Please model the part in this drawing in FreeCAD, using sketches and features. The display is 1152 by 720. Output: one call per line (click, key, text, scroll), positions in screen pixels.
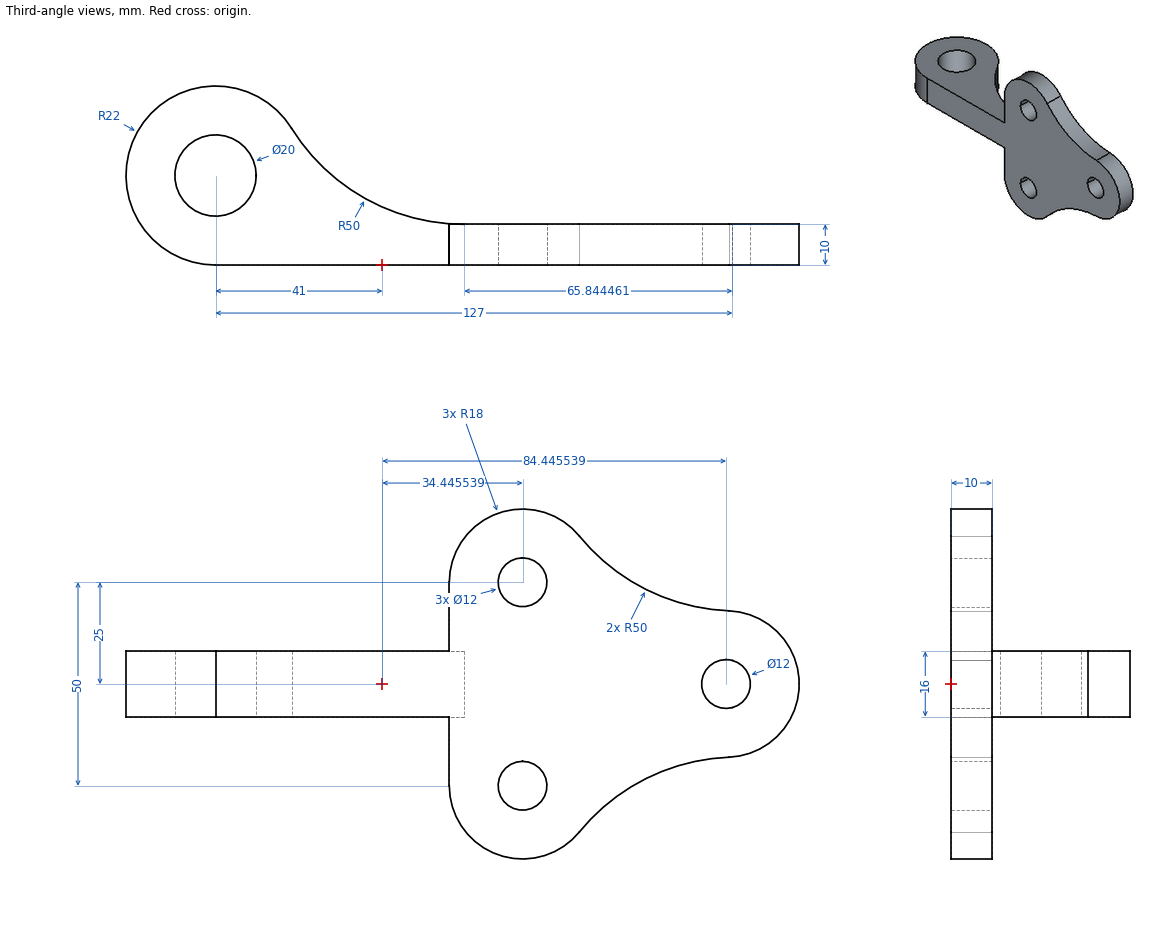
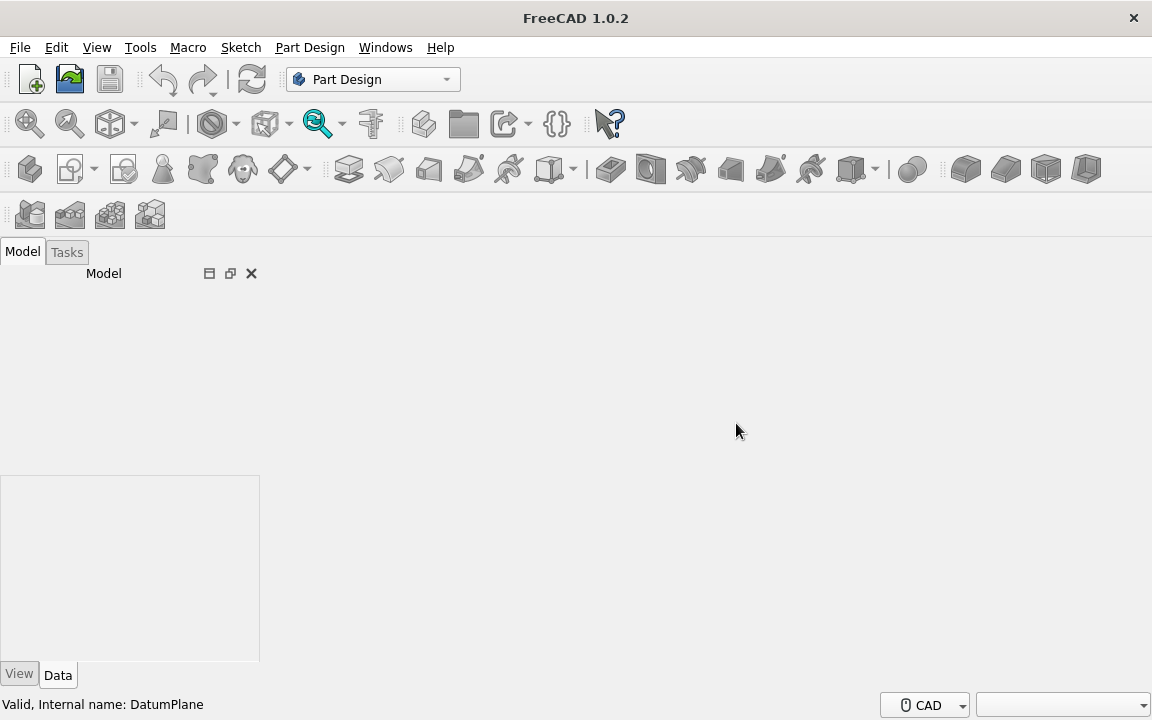
key(ctrl+n)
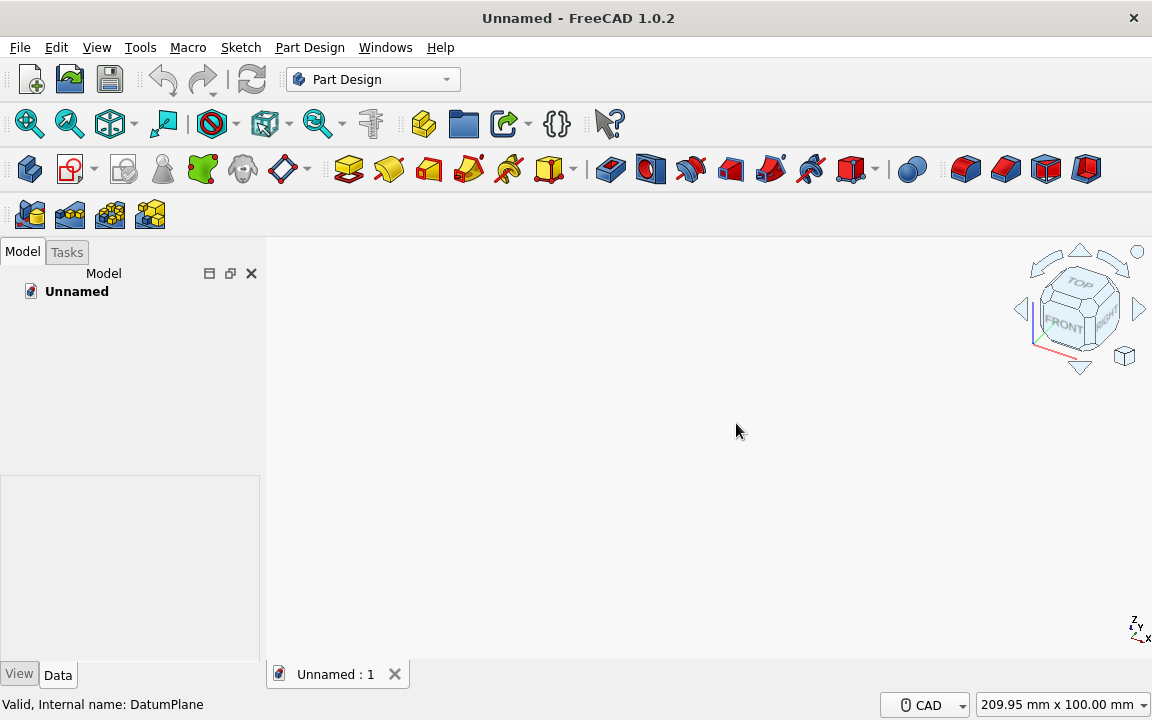
click(70, 170)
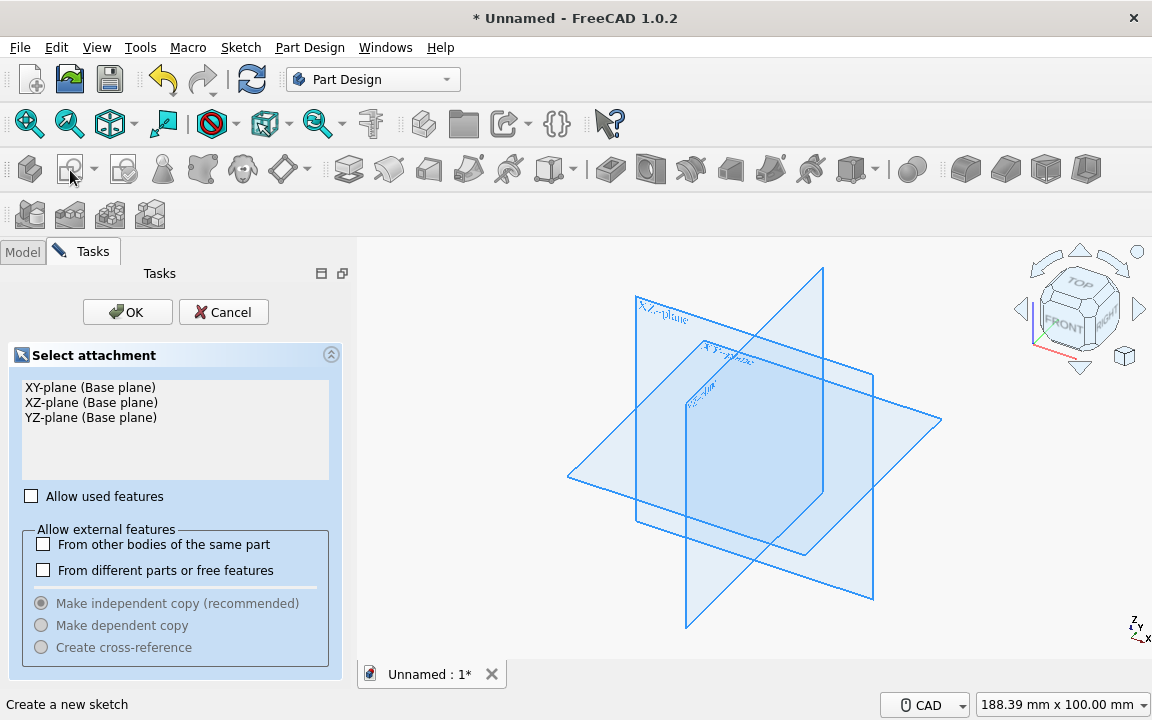
click(82, 388)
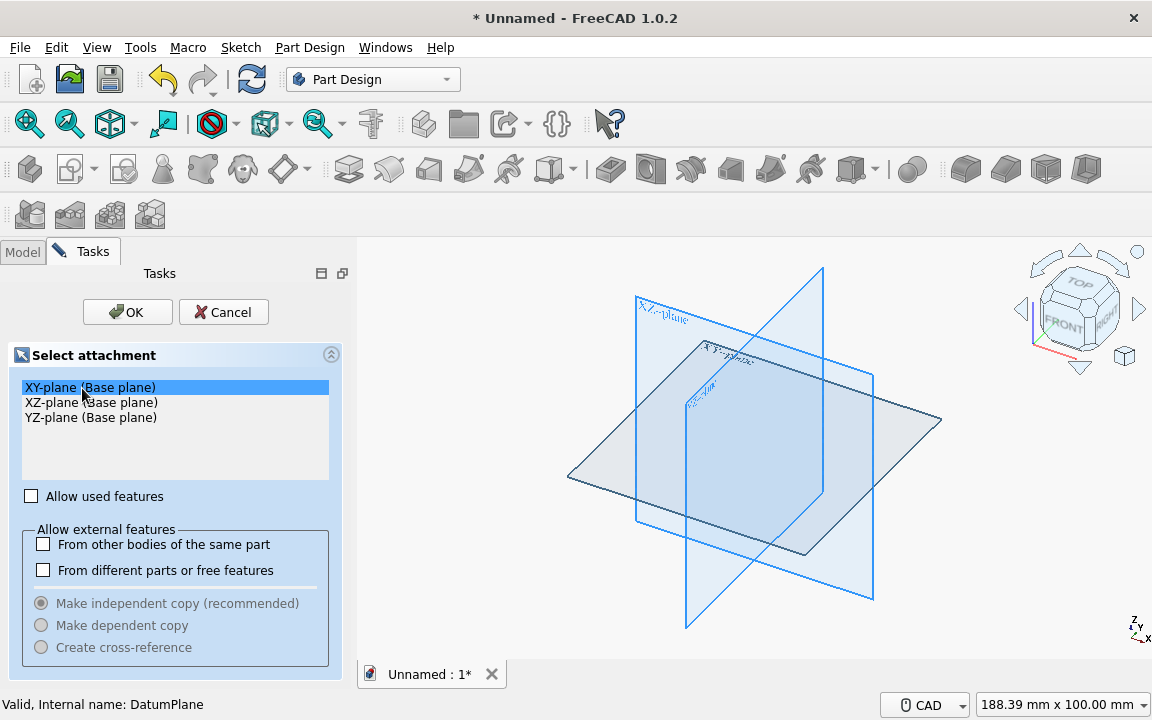
click(128, 312)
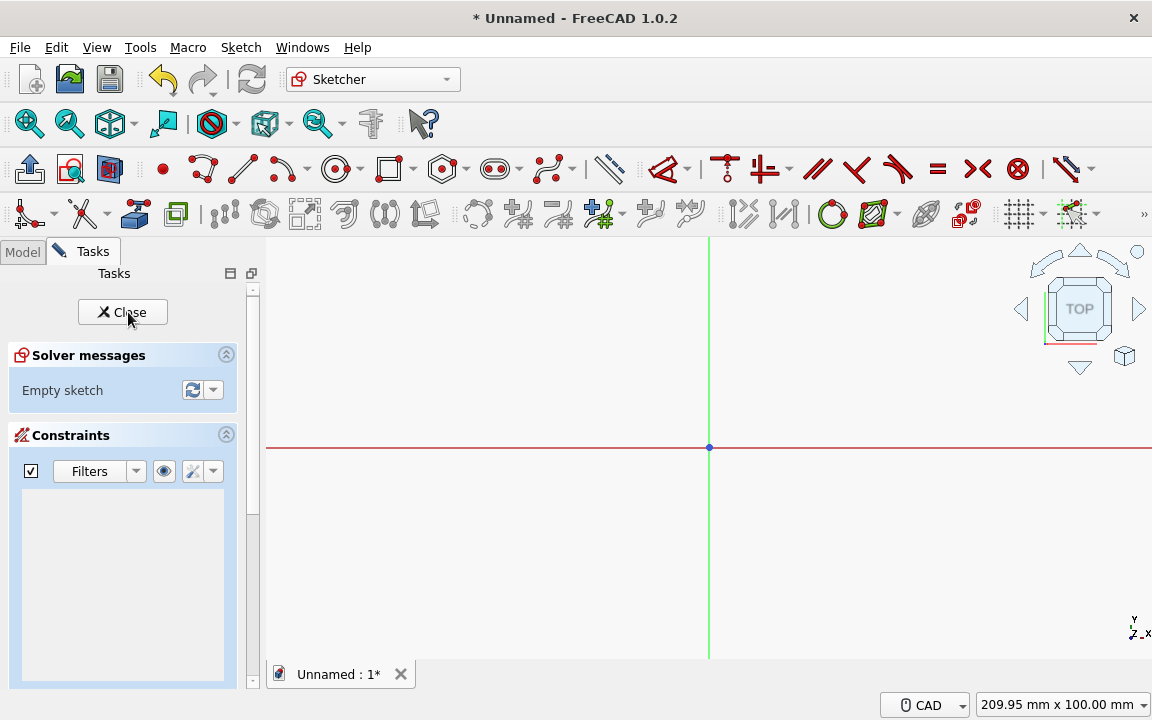
scroll(294, 631, down, 1)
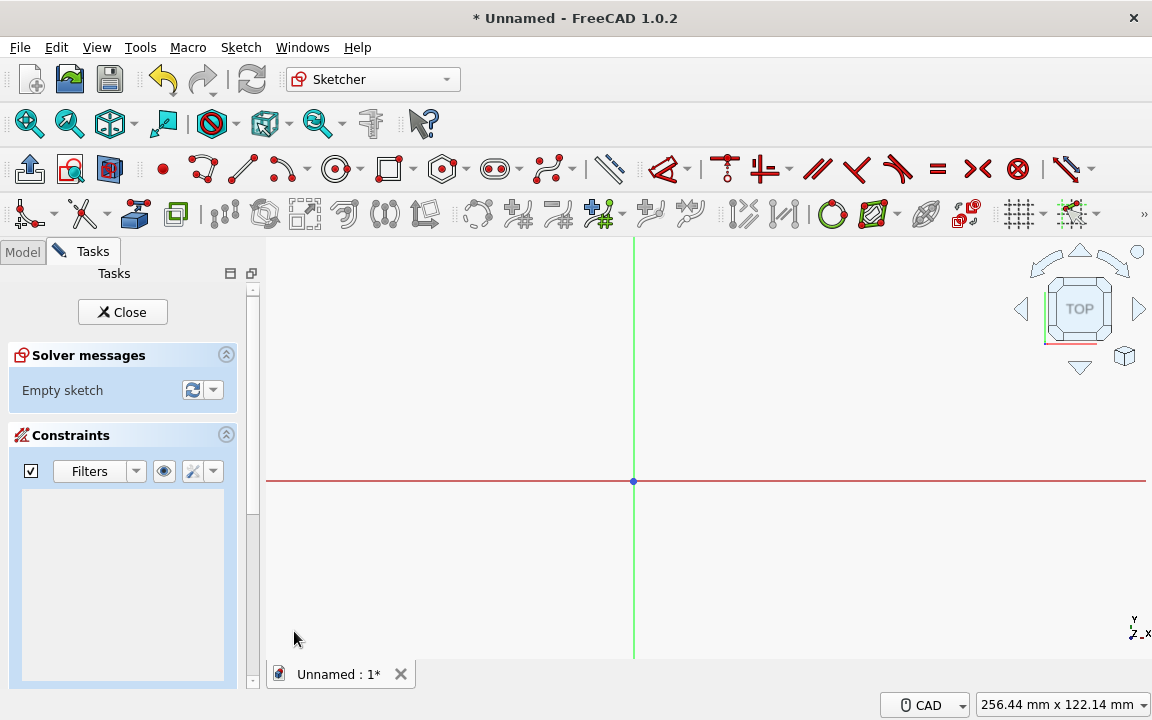
key(g)
key(m)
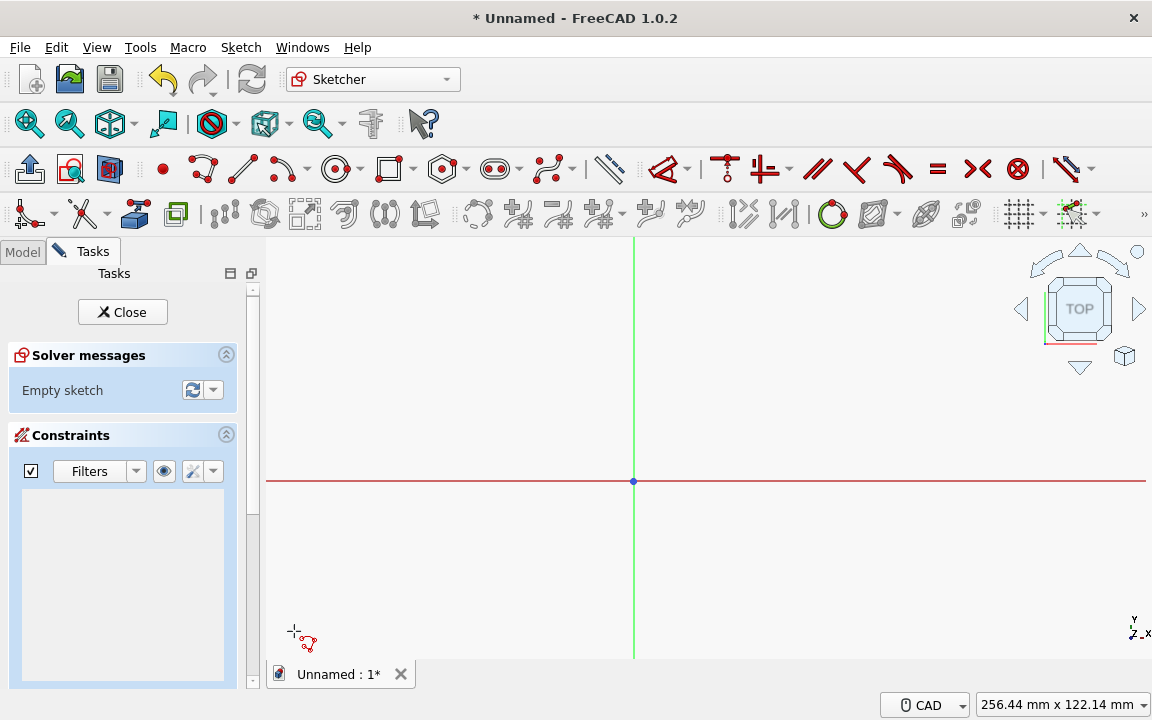
click(492, 481)
click(931, 472)
click(931, 447)
click(703, 447)
right_click(703, 447)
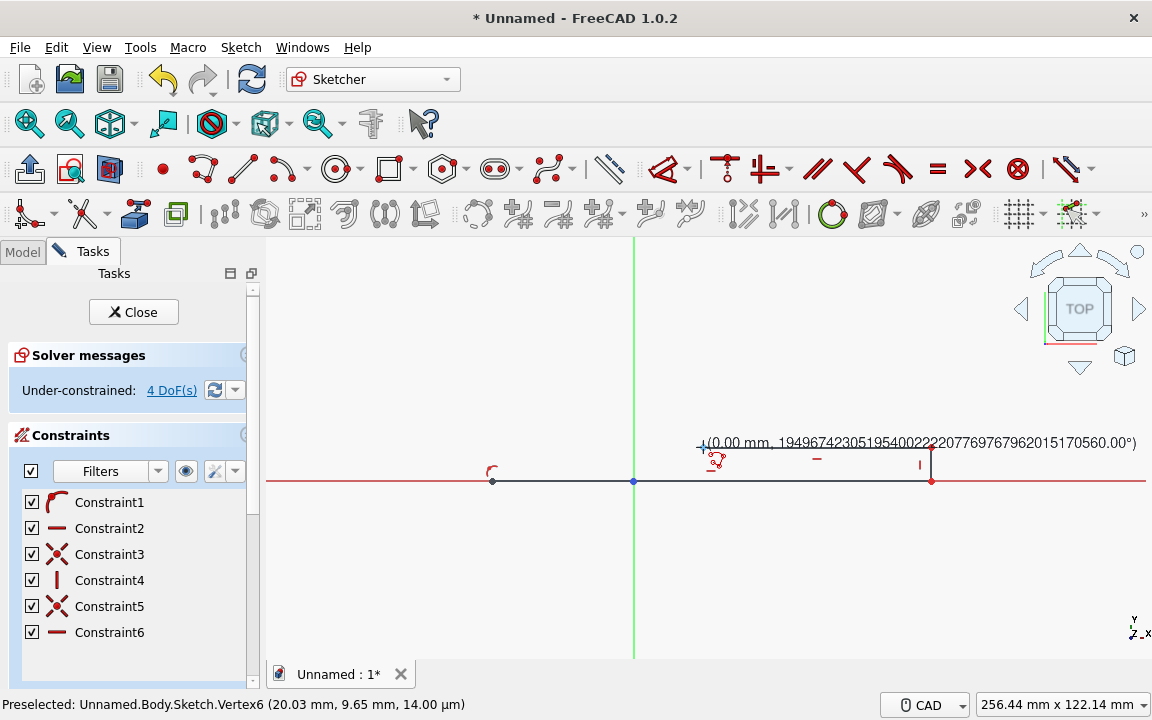
key(g)
key(3)
key(a)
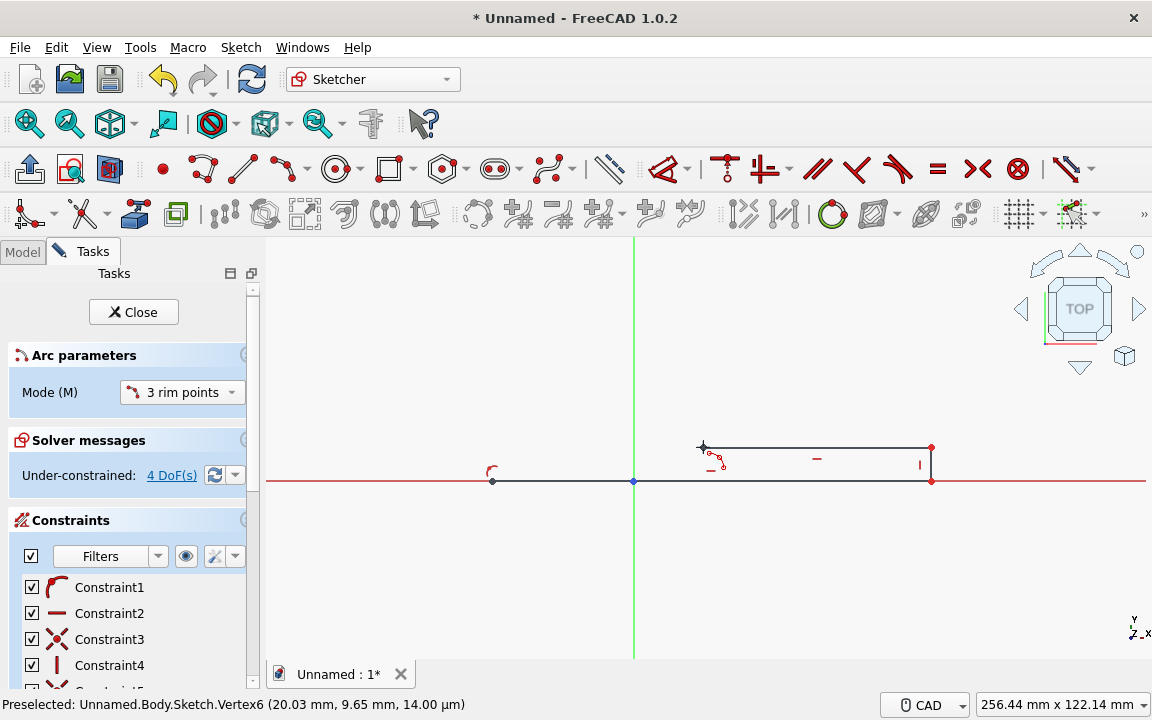
click(703, 448)
click(557, 365)
click(619, 425)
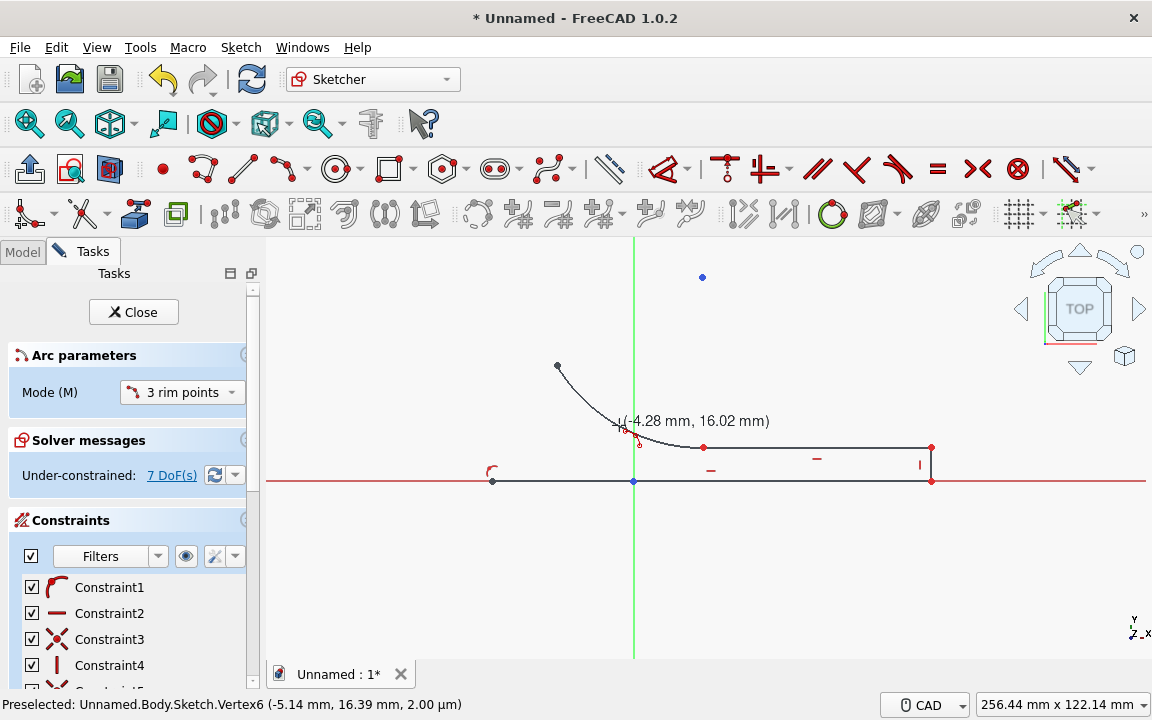
click(557, 366)
click(492, 481)
click(426, 368)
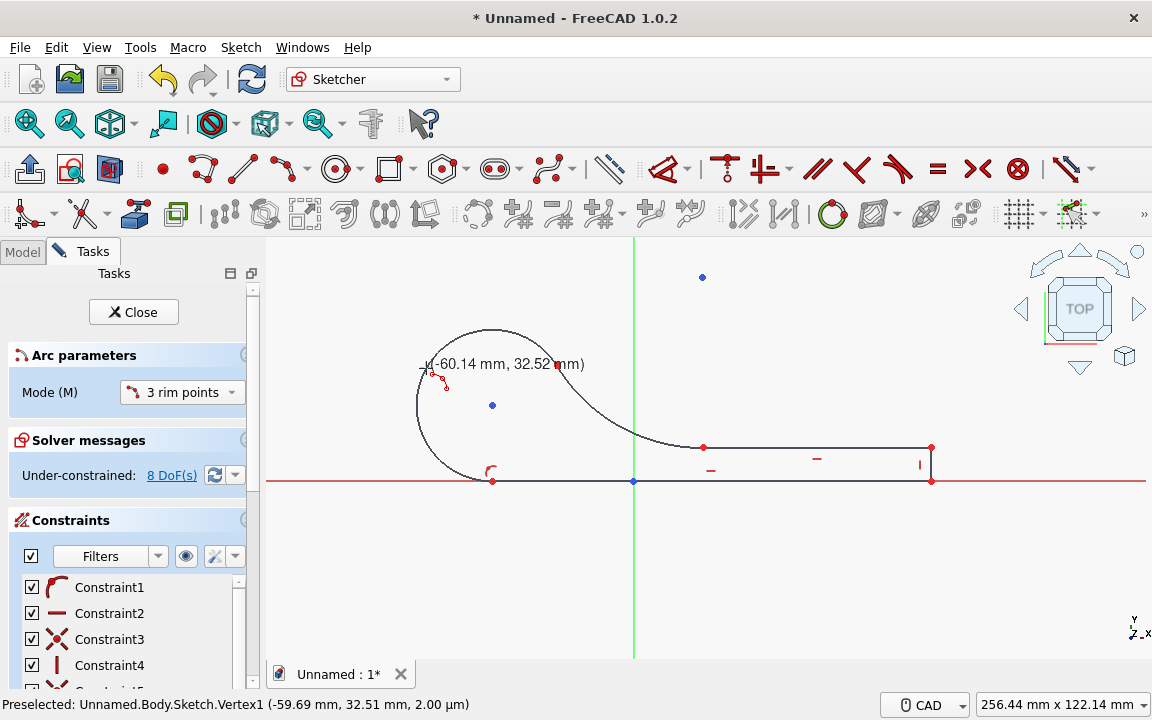
key(g)
key(c)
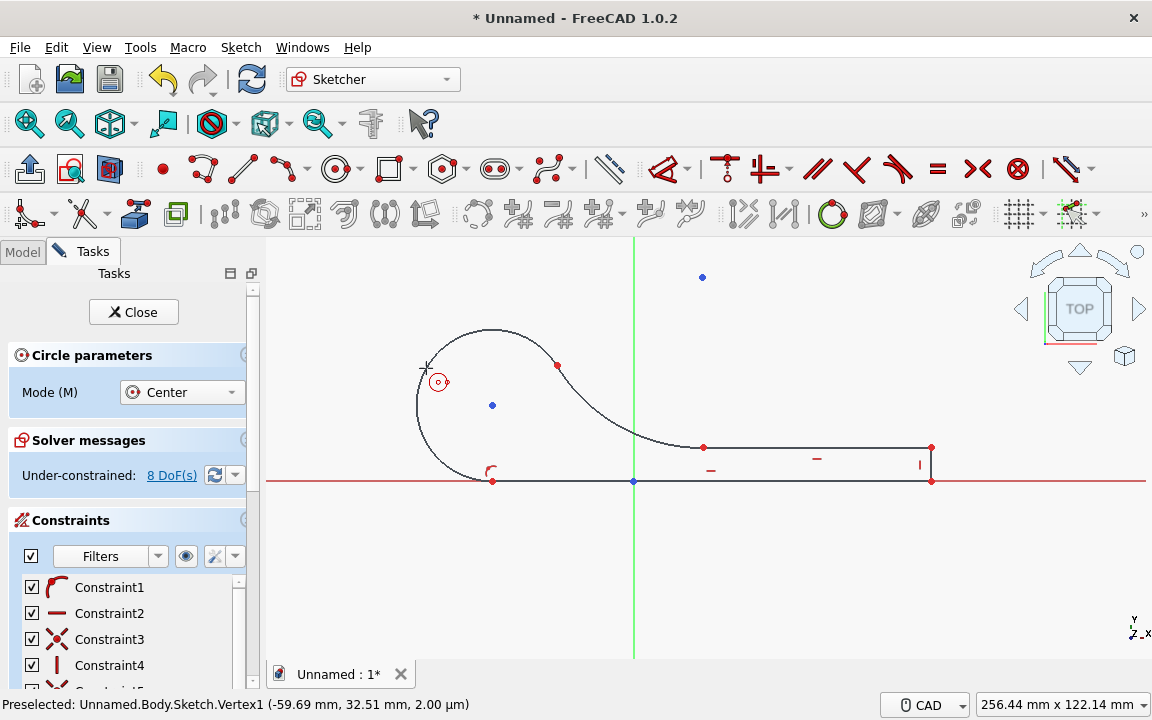
click(492, 405)
click(517, 381)
key(Escape)